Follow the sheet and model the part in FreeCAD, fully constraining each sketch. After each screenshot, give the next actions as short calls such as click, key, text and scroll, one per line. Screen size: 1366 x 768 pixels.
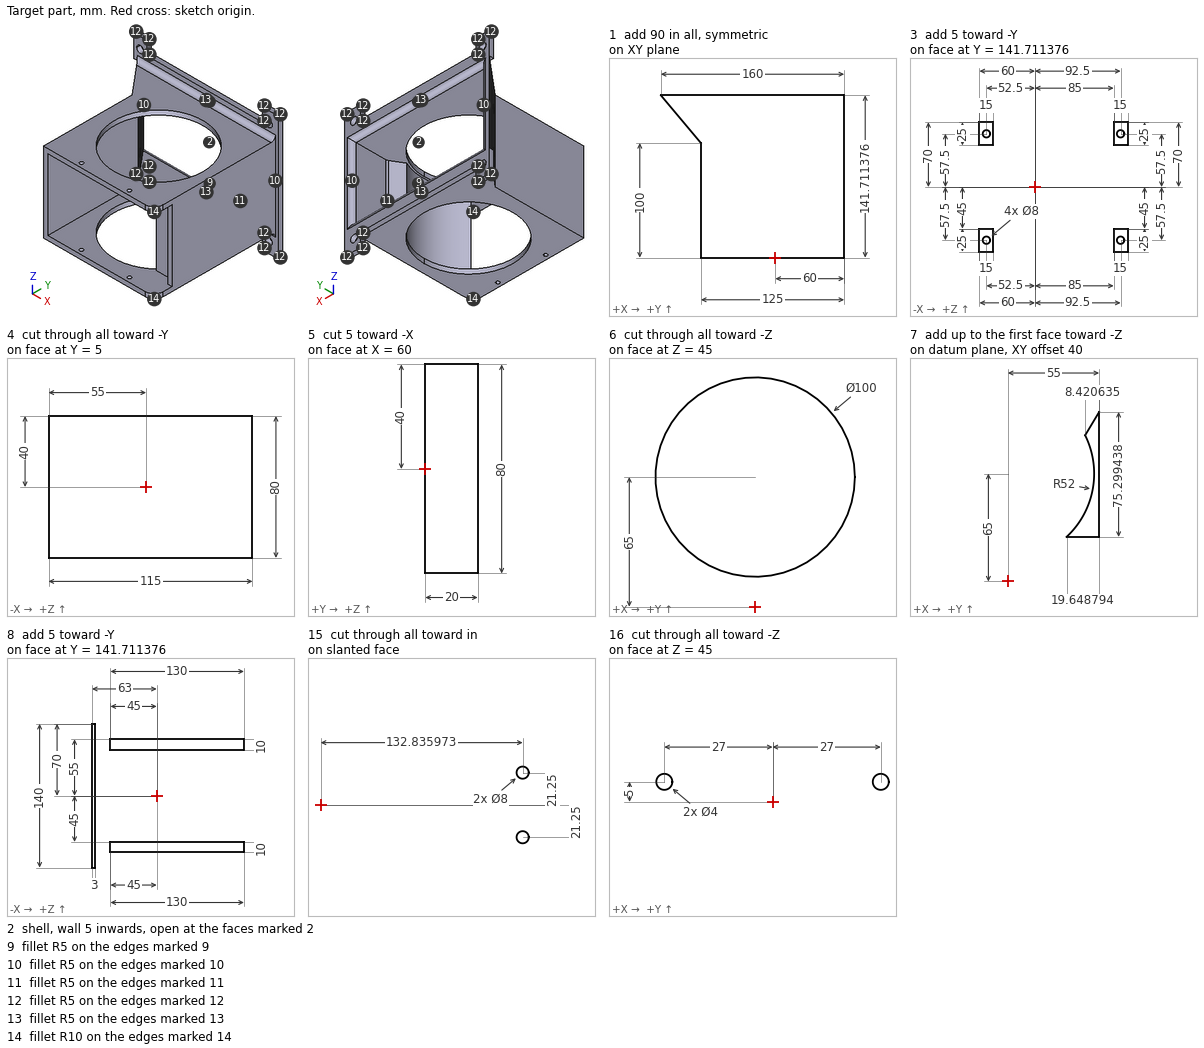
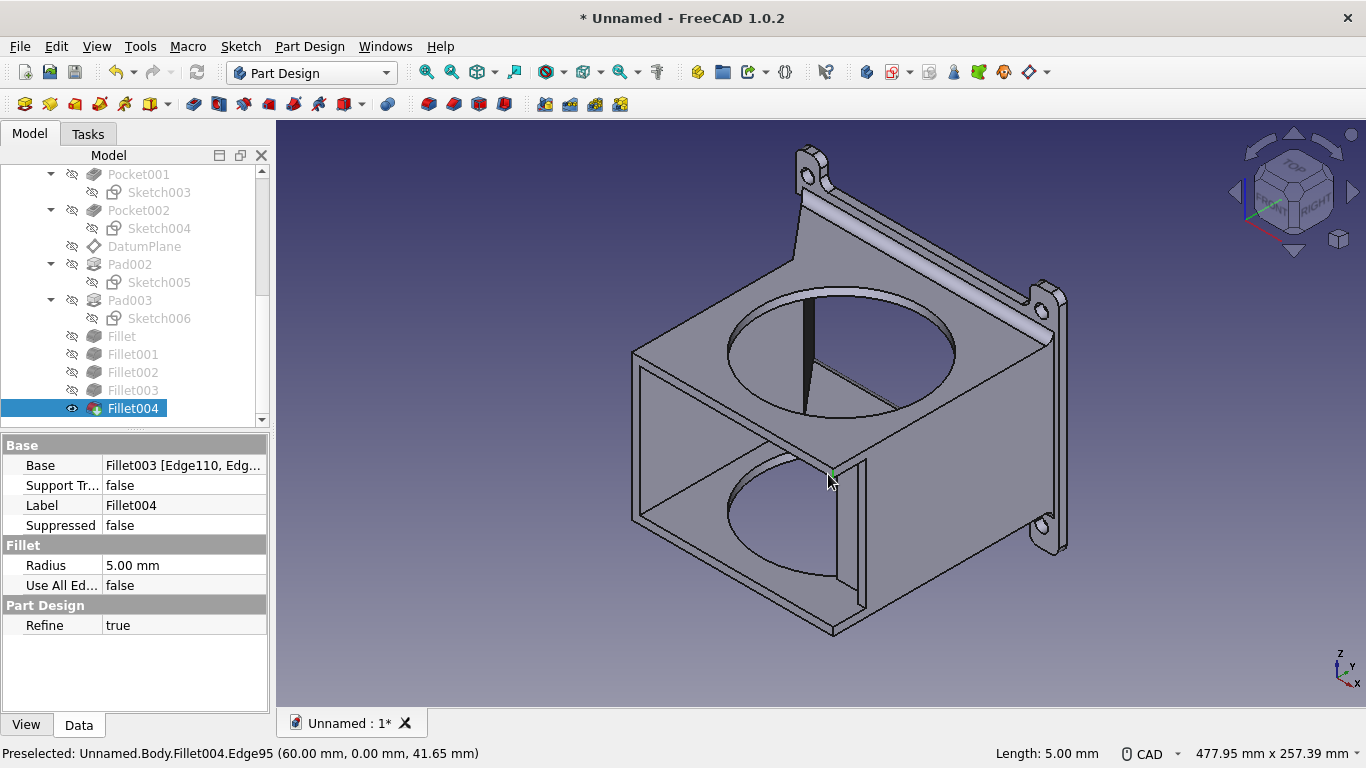
click(833, 632, ctrl)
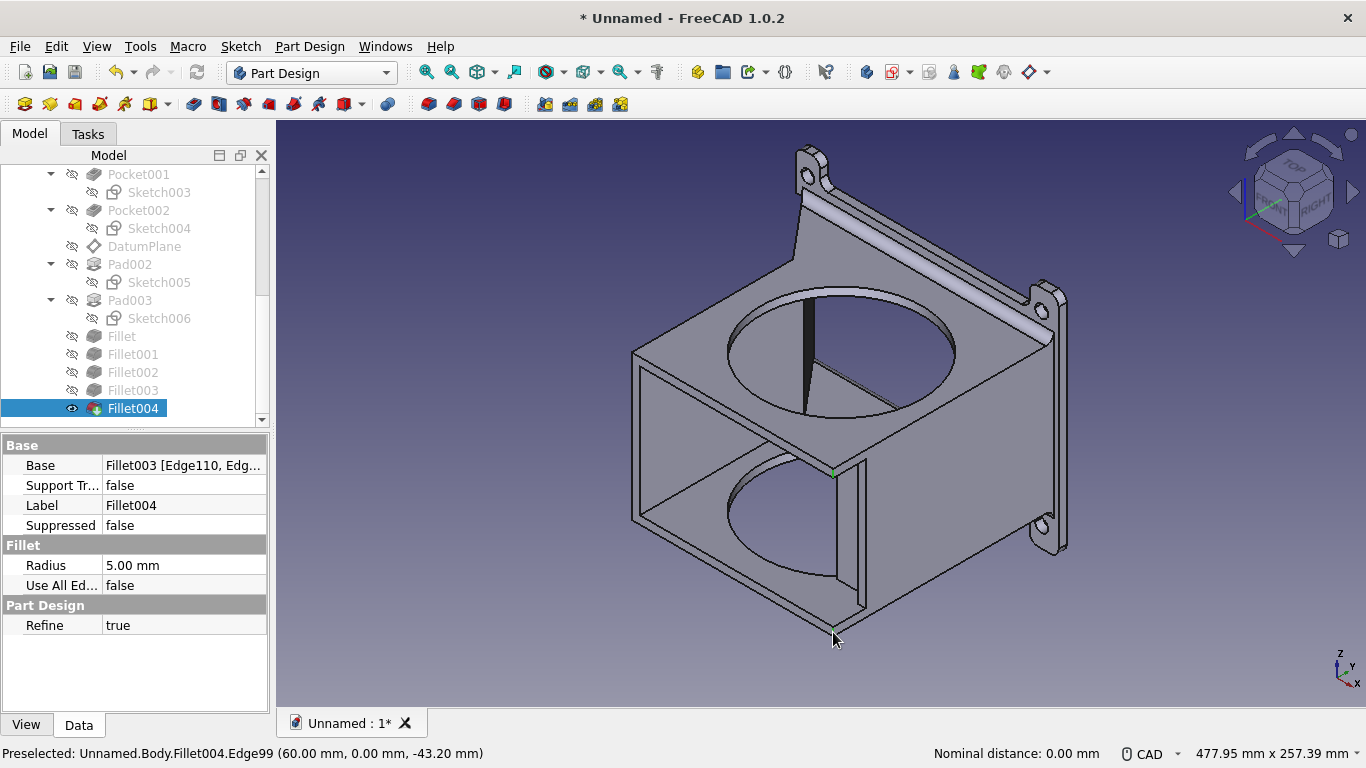
click(429, 104)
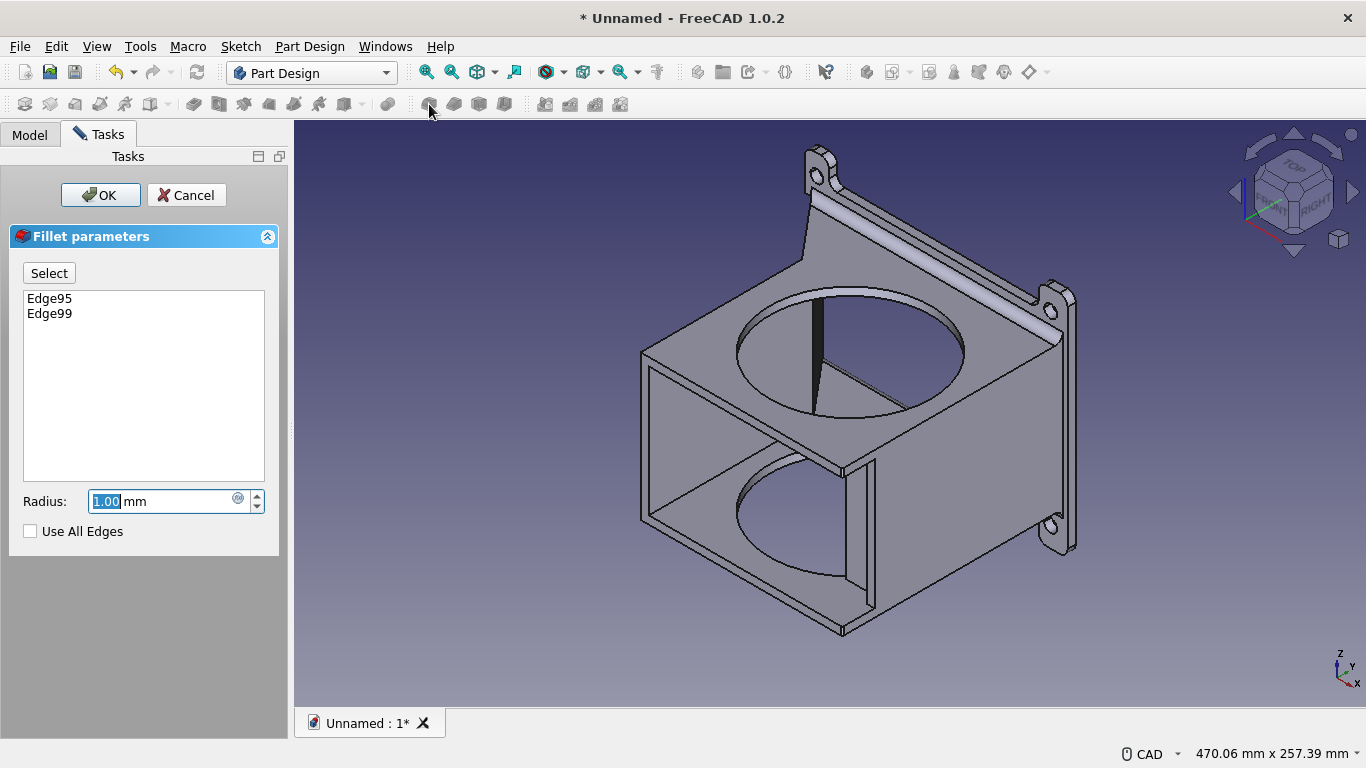
text(10)
key(Tab)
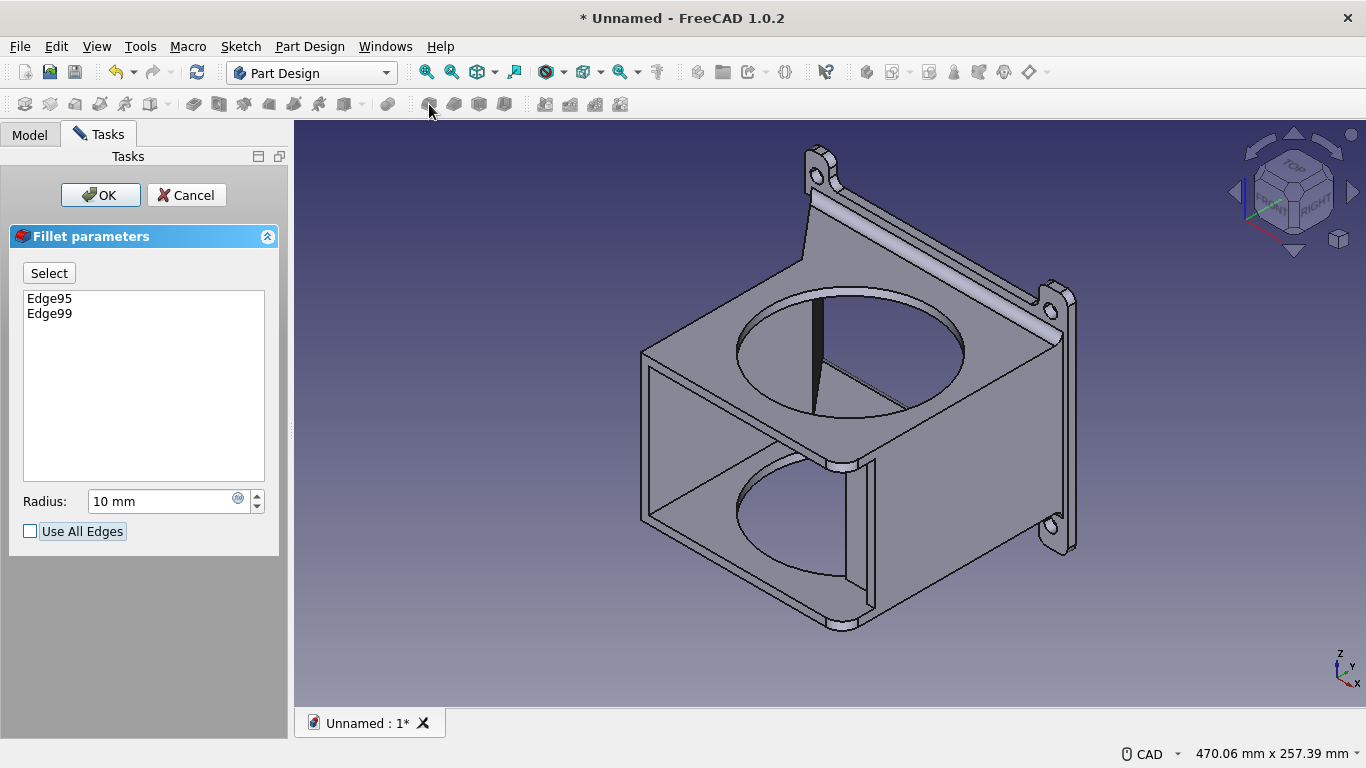
click(101, 195)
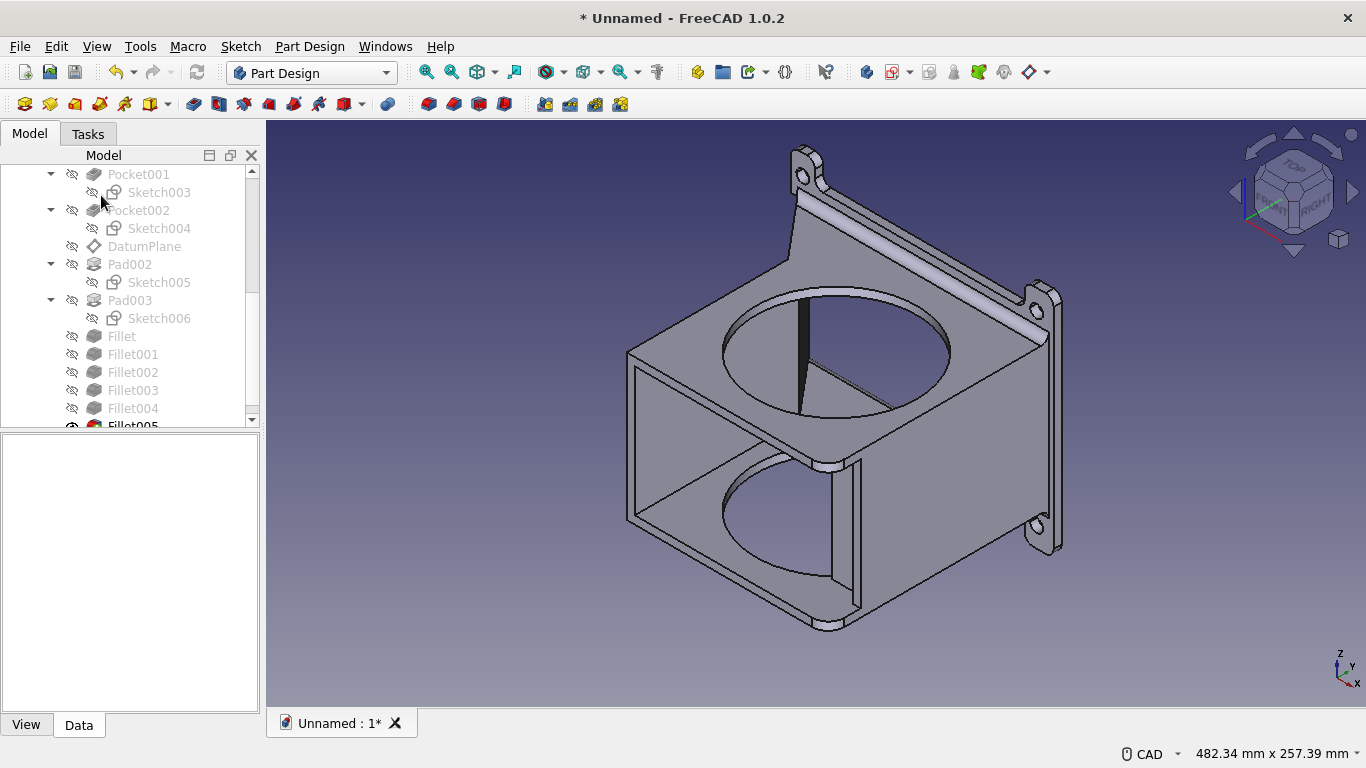
key(3)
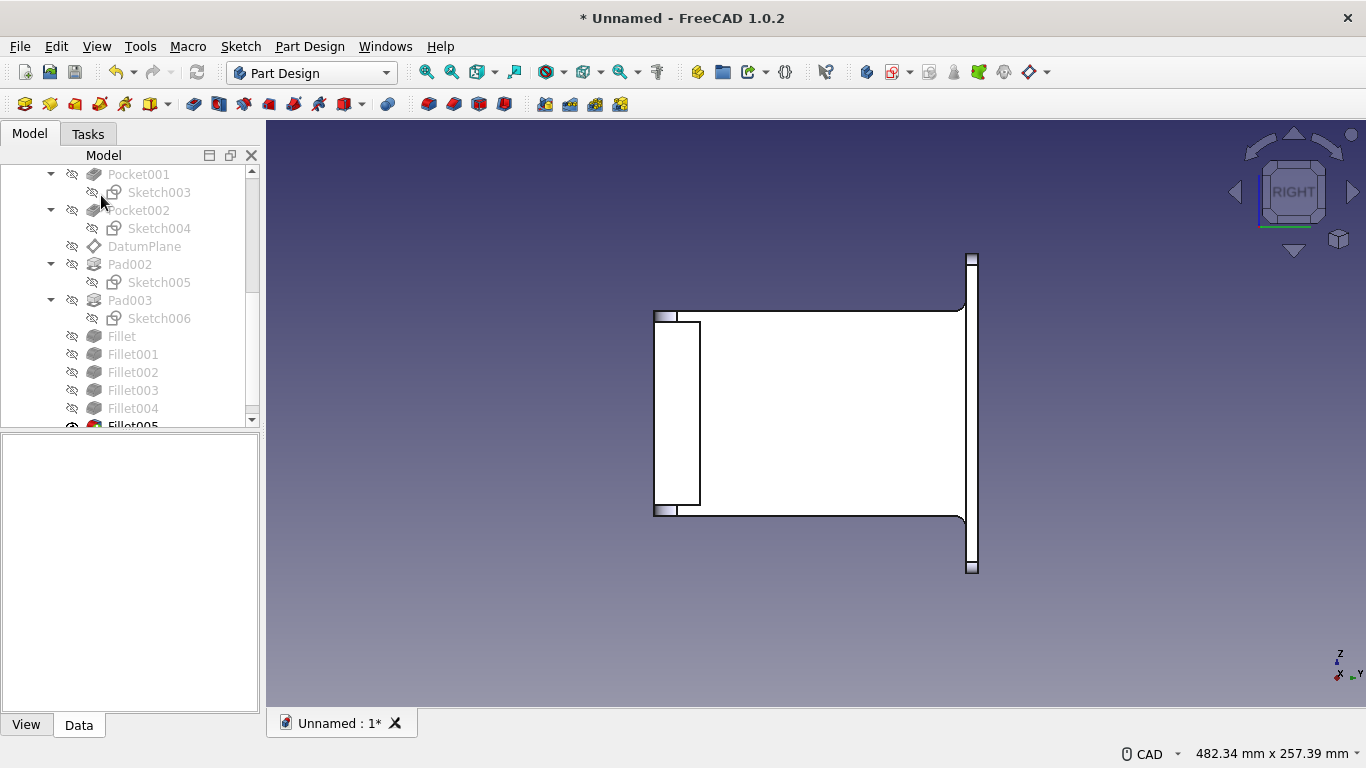
key(4)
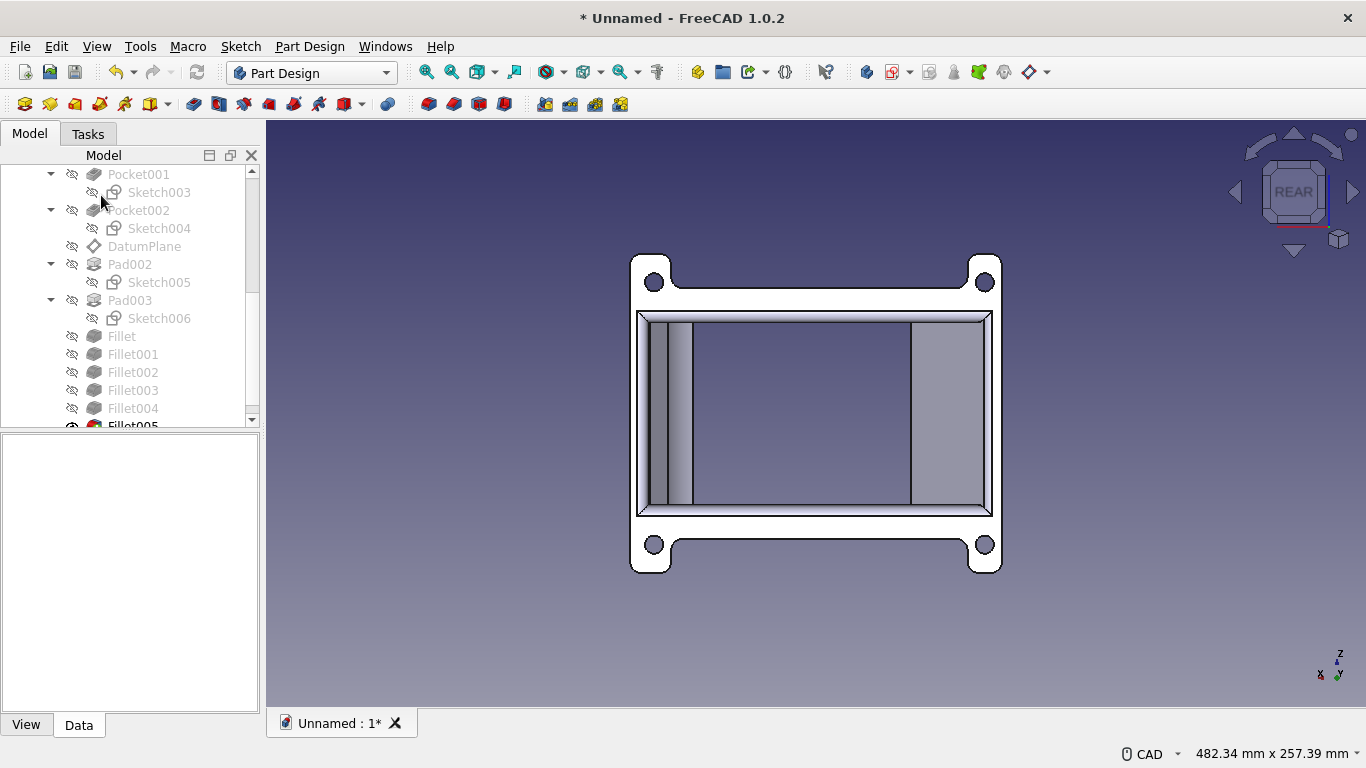
click(947, 386)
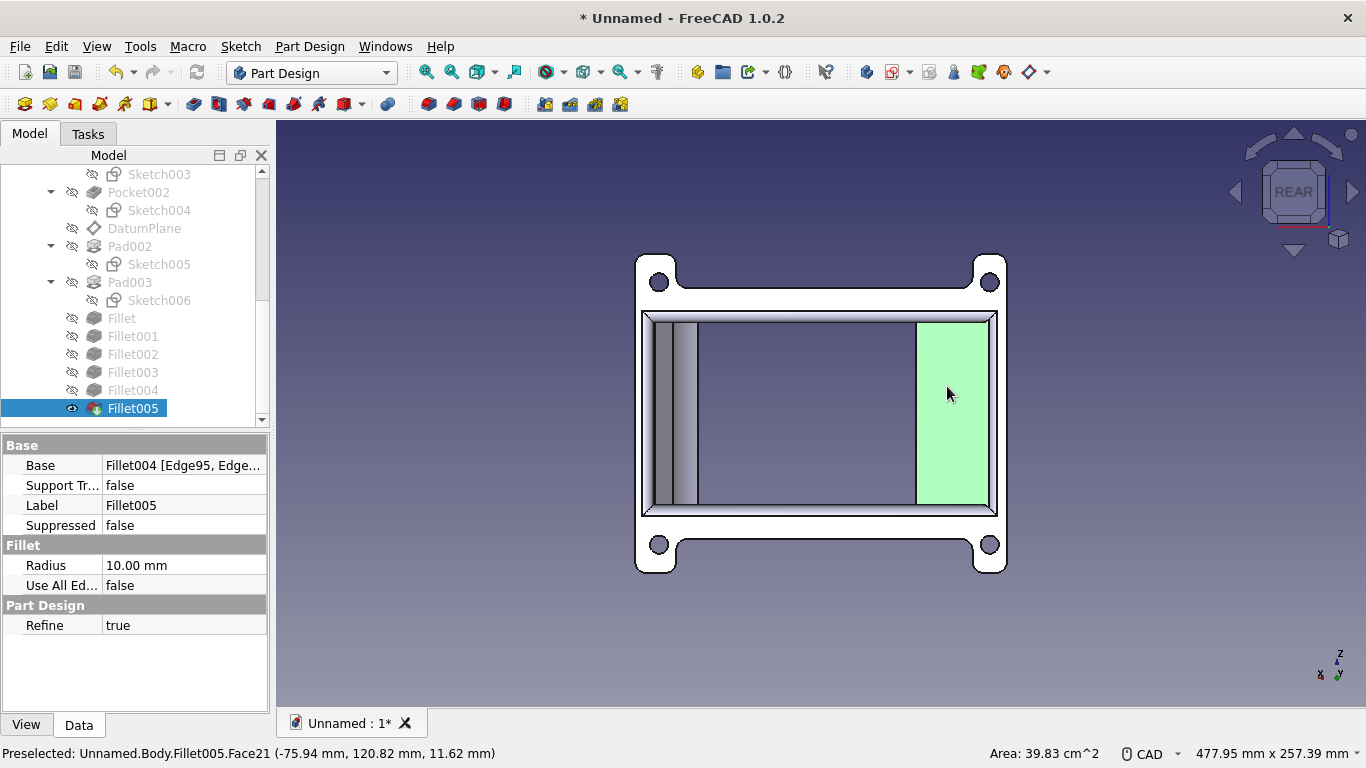
click(892, 72)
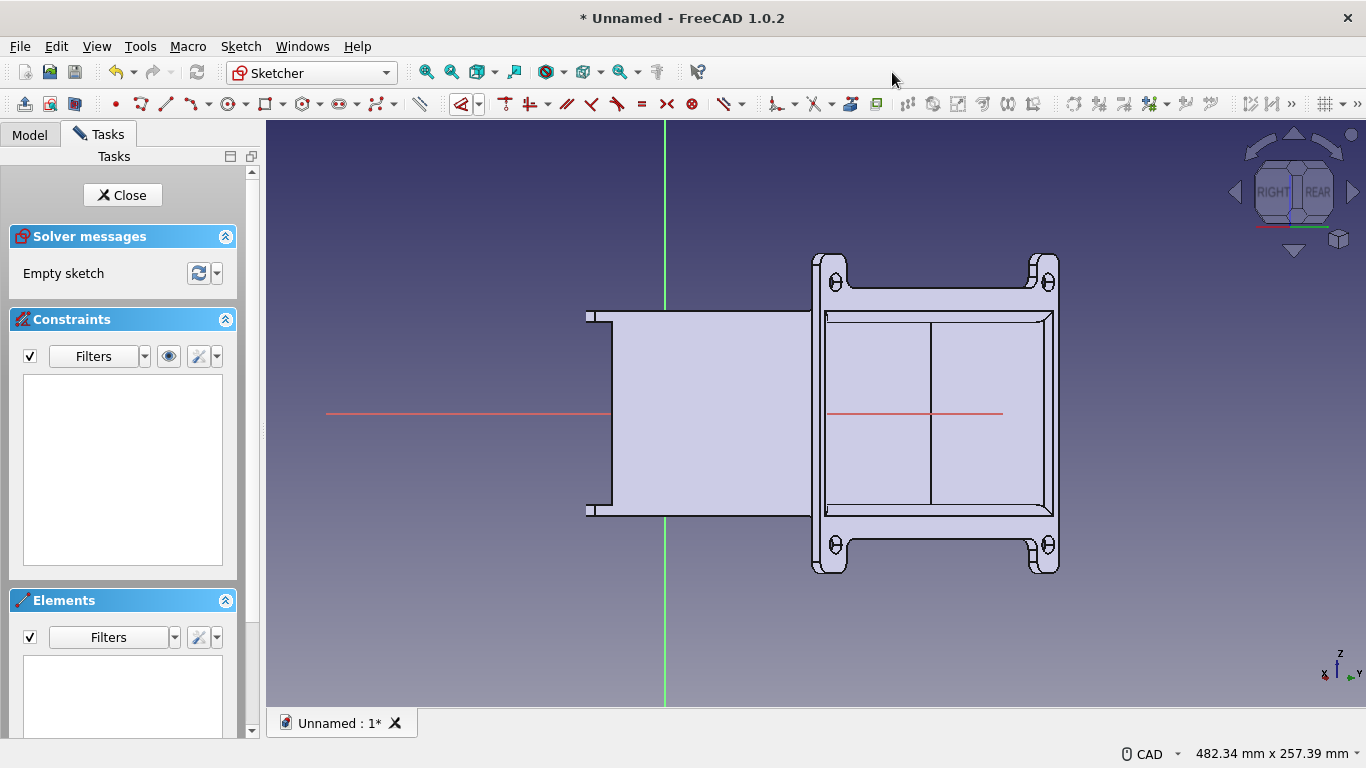
key(q)
key(s)